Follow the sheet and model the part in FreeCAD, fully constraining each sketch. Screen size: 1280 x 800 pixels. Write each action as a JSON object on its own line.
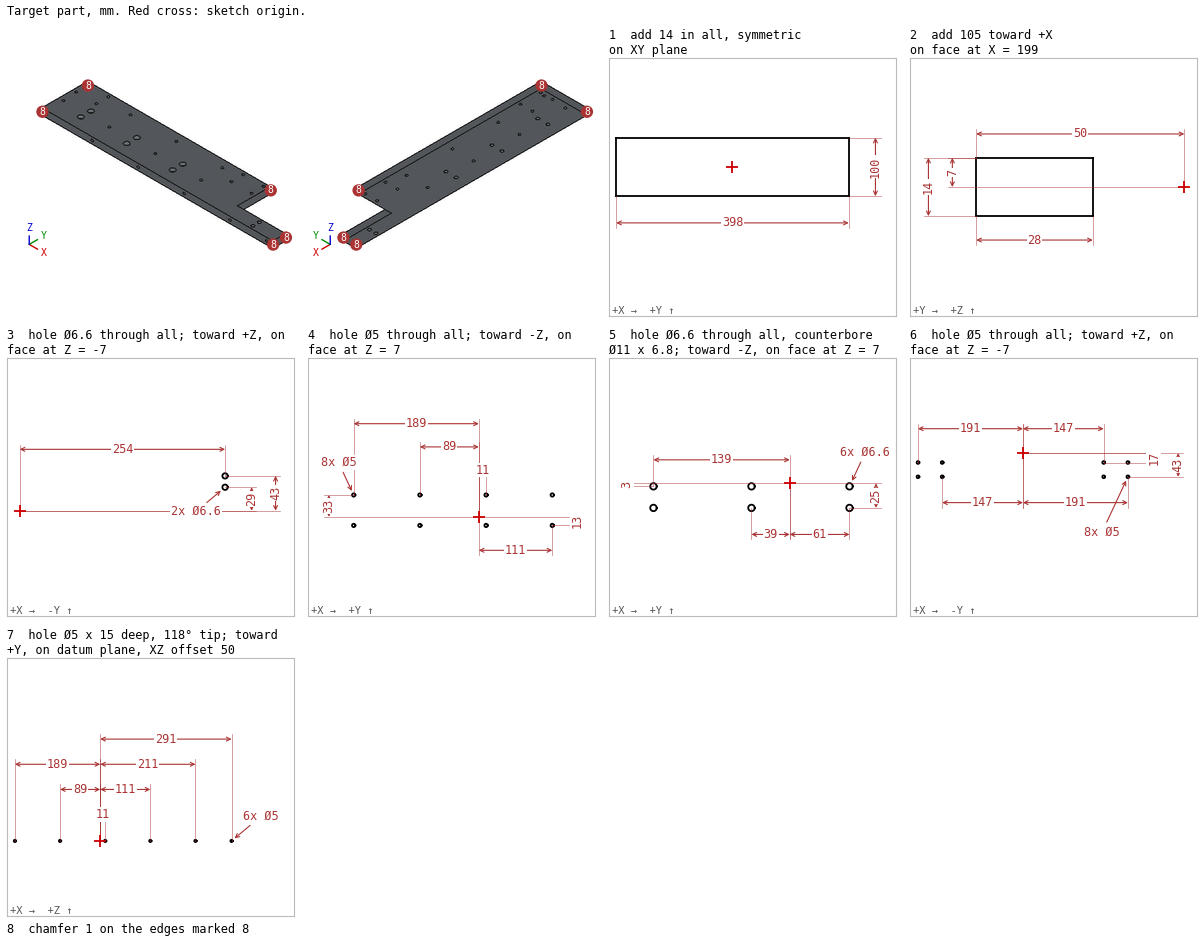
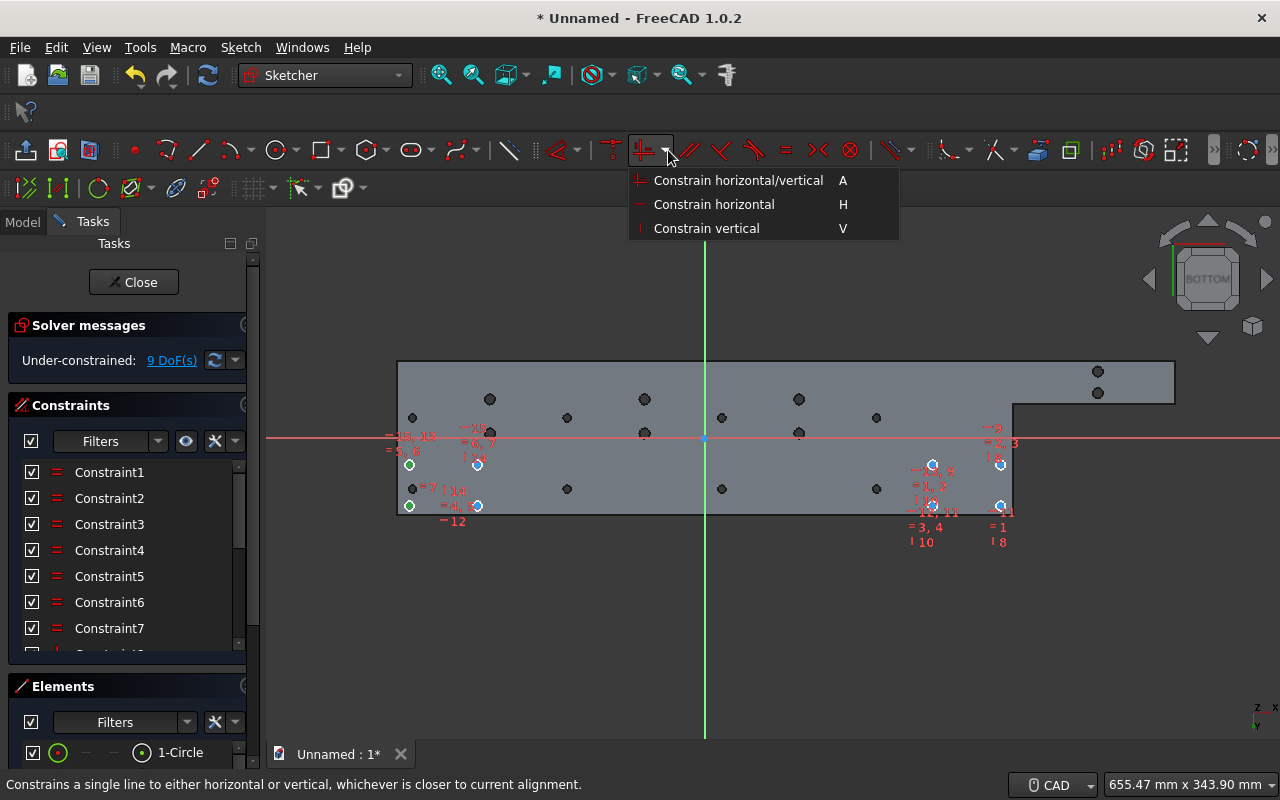
{"action": "left_click", "coordinate": [764, 228]}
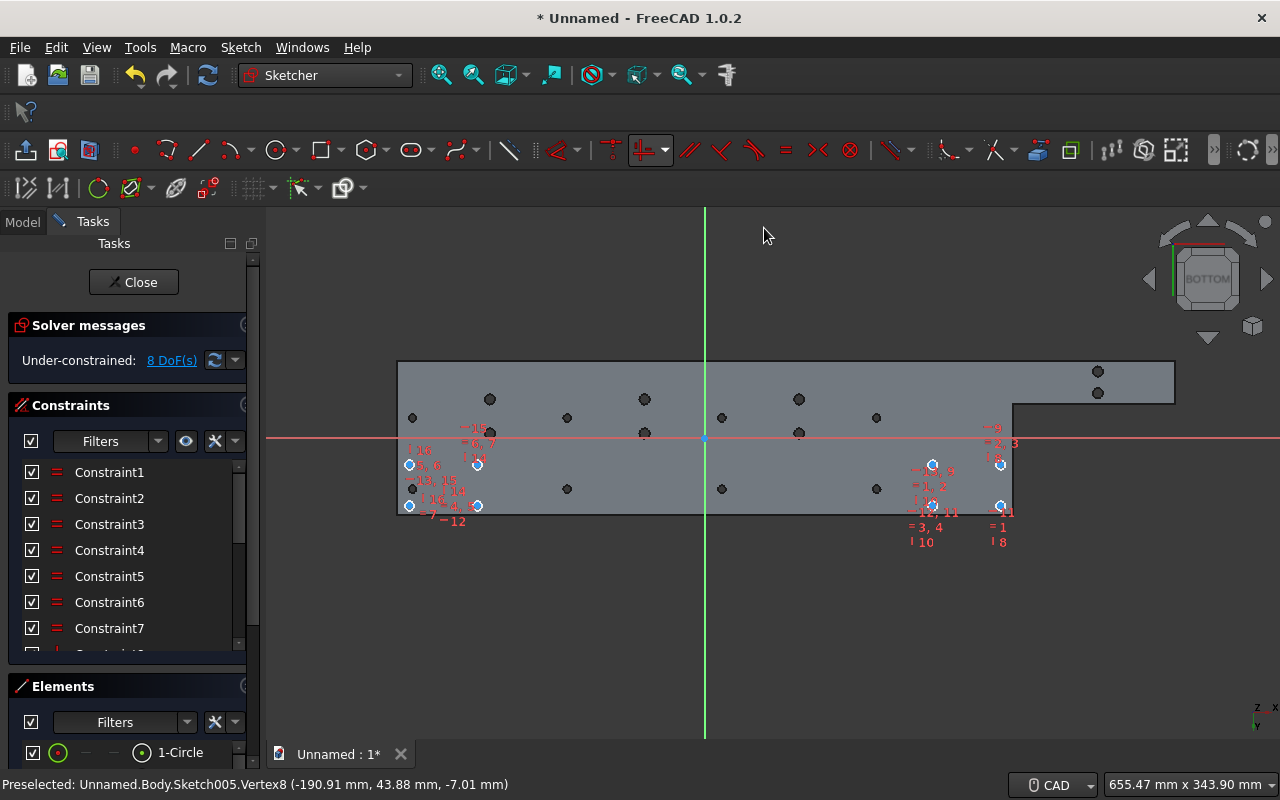
{"action": "left_click", "coordinate": [478, 506]}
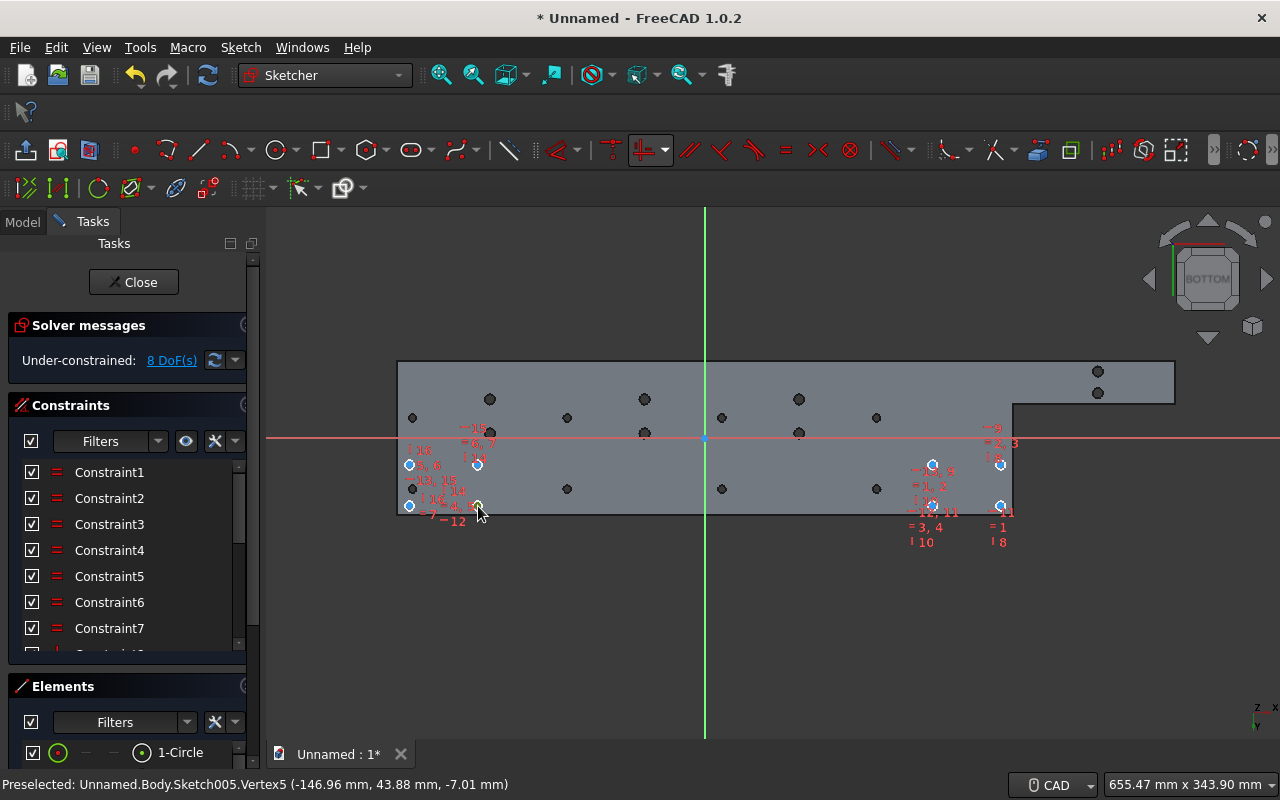
{"action": "left_click", "coordinate": [410, 506]}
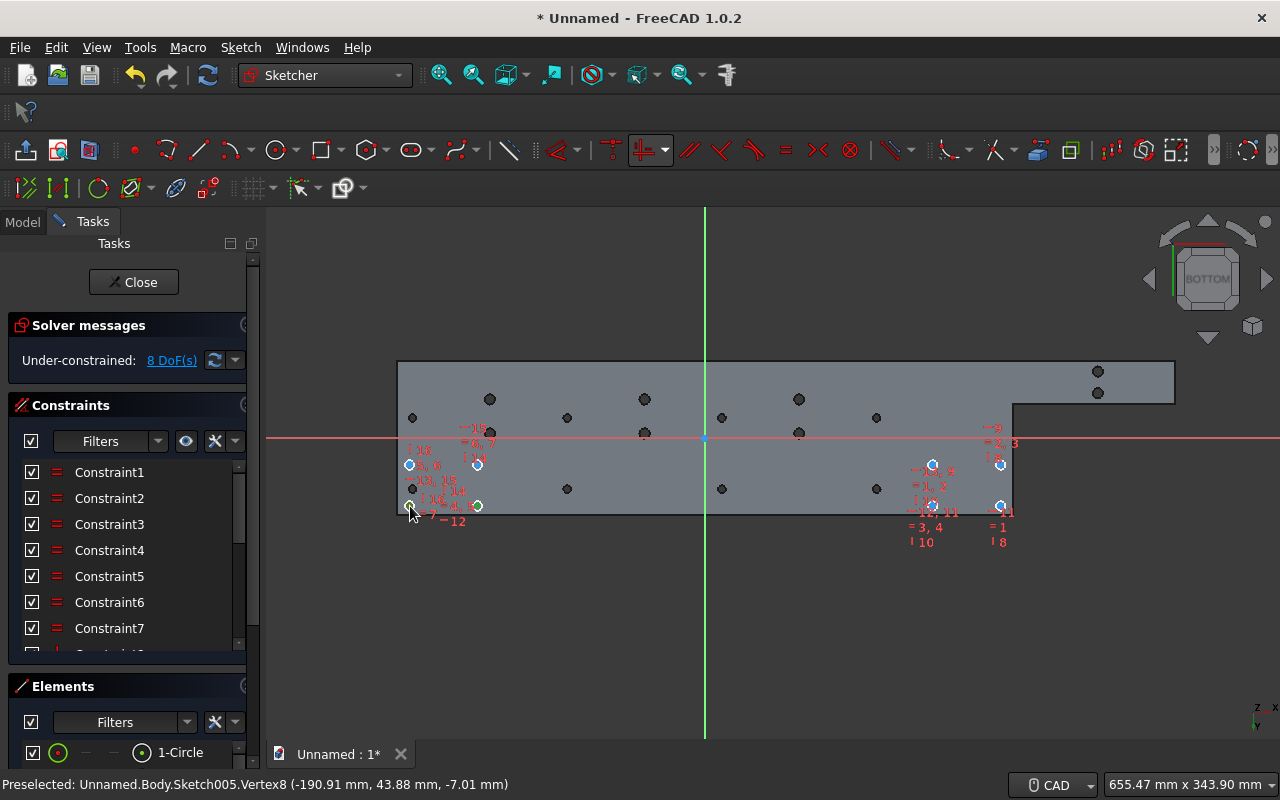
{"action": "key", "text": "h"}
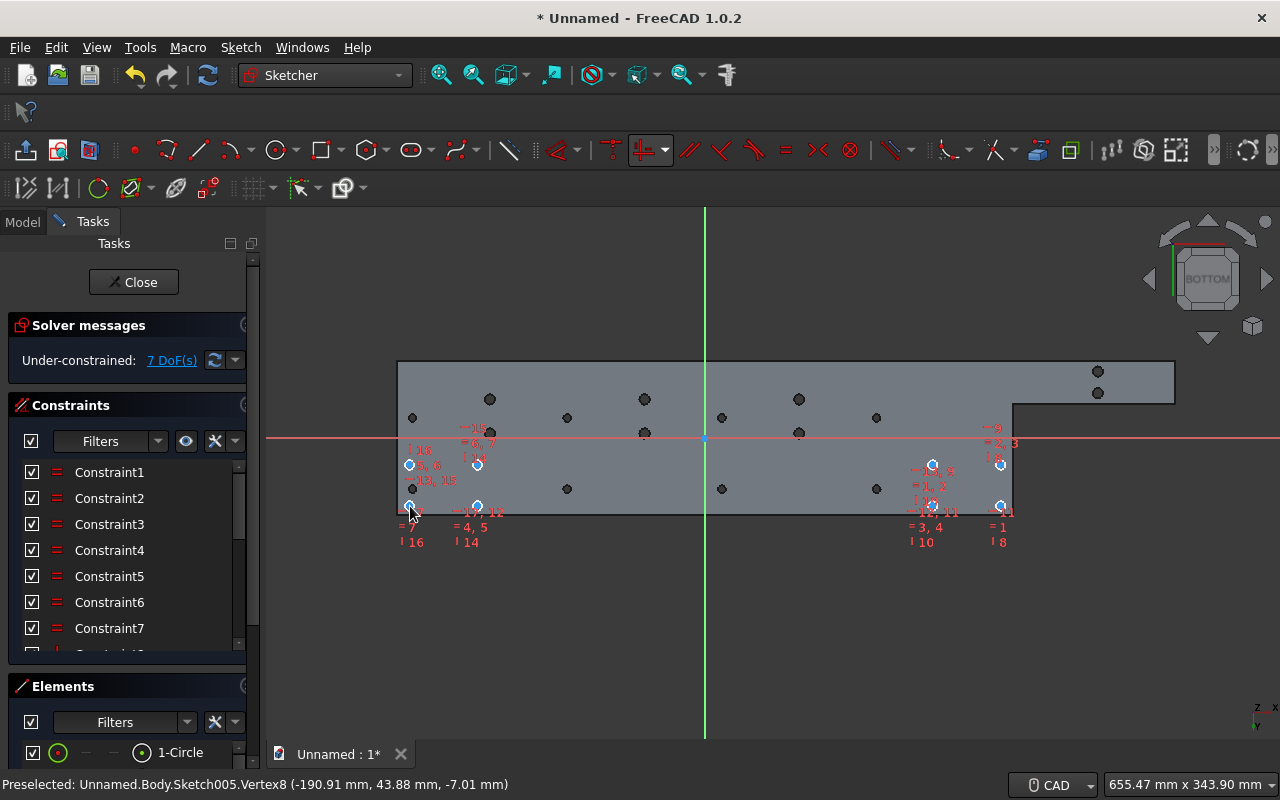
{"action": "key", "text": "d"}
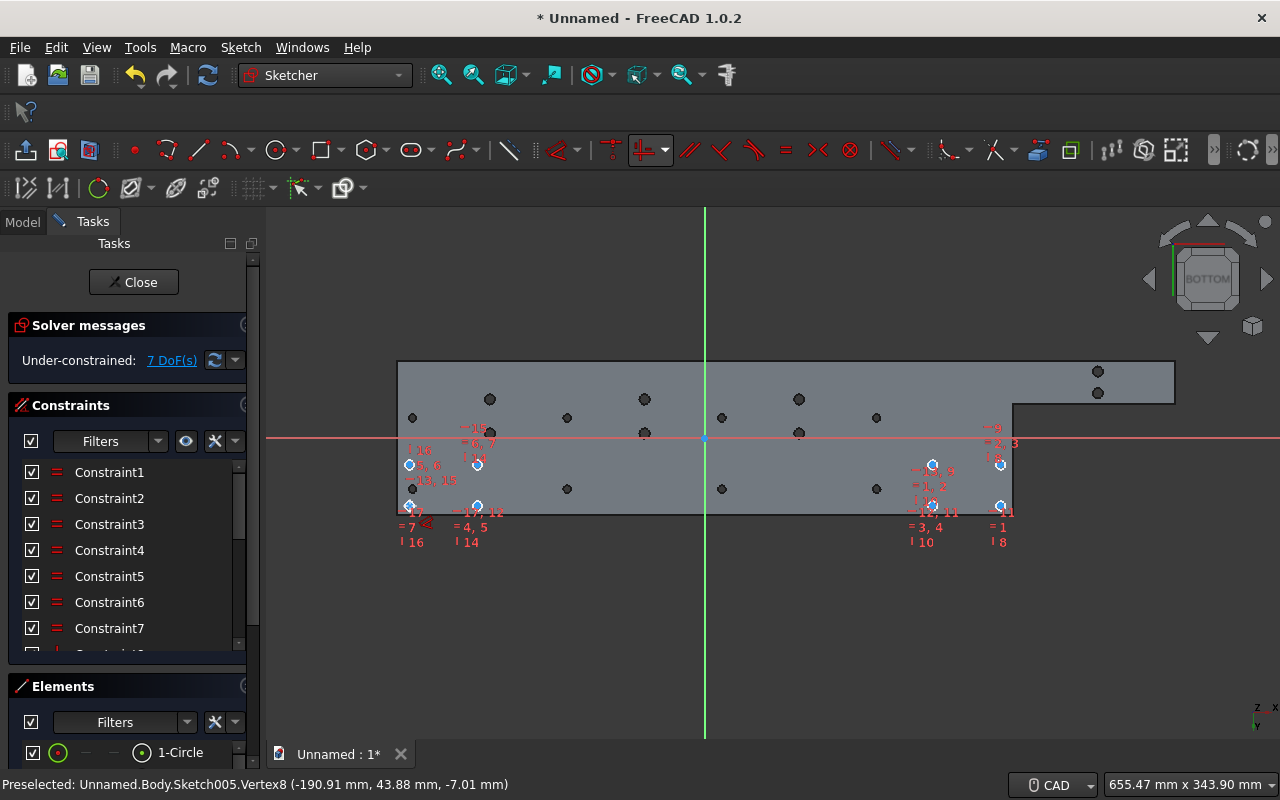
{"action": "scroll", "coordinate": [1004, 503], "scroll_direction": "up", "scroll_amount": 9}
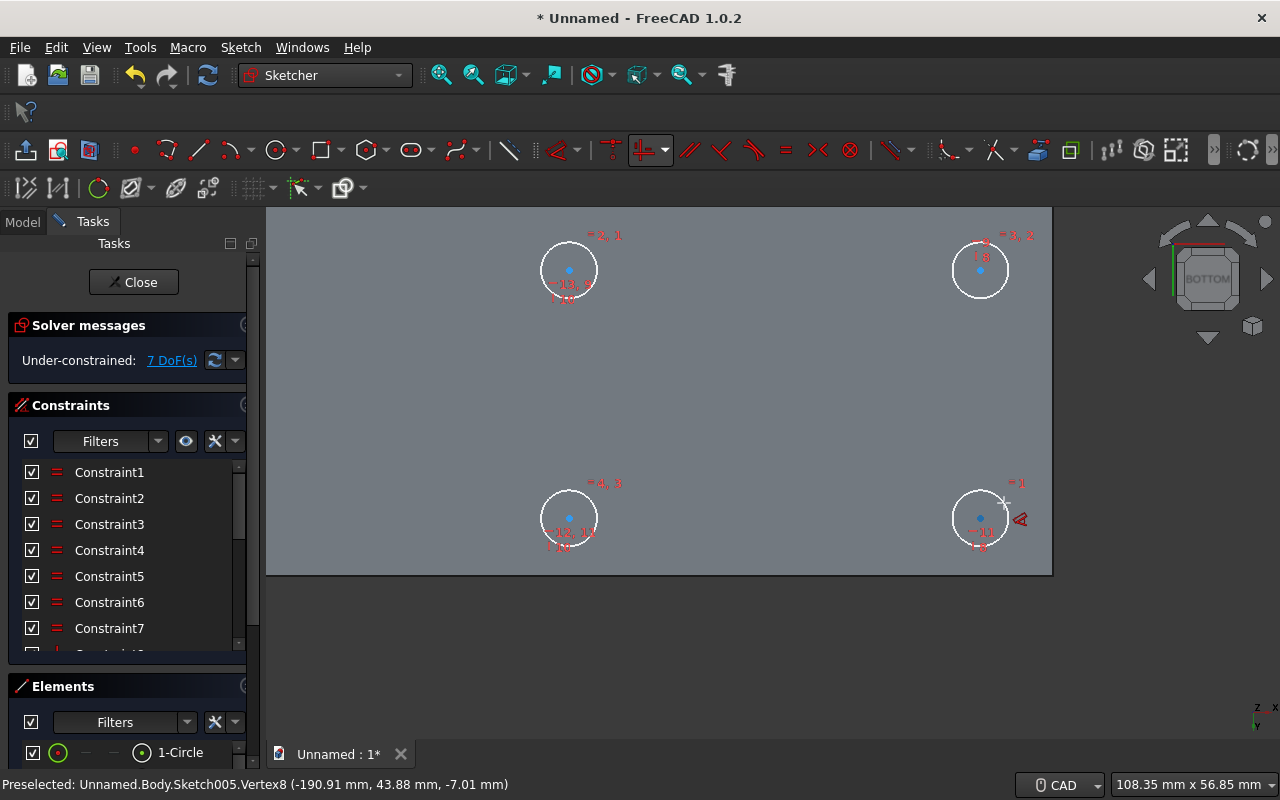
{"action": "left_click", "coordinate": [1000, 499]}
{"action": "left_click", "coordinate": [1023, 476]}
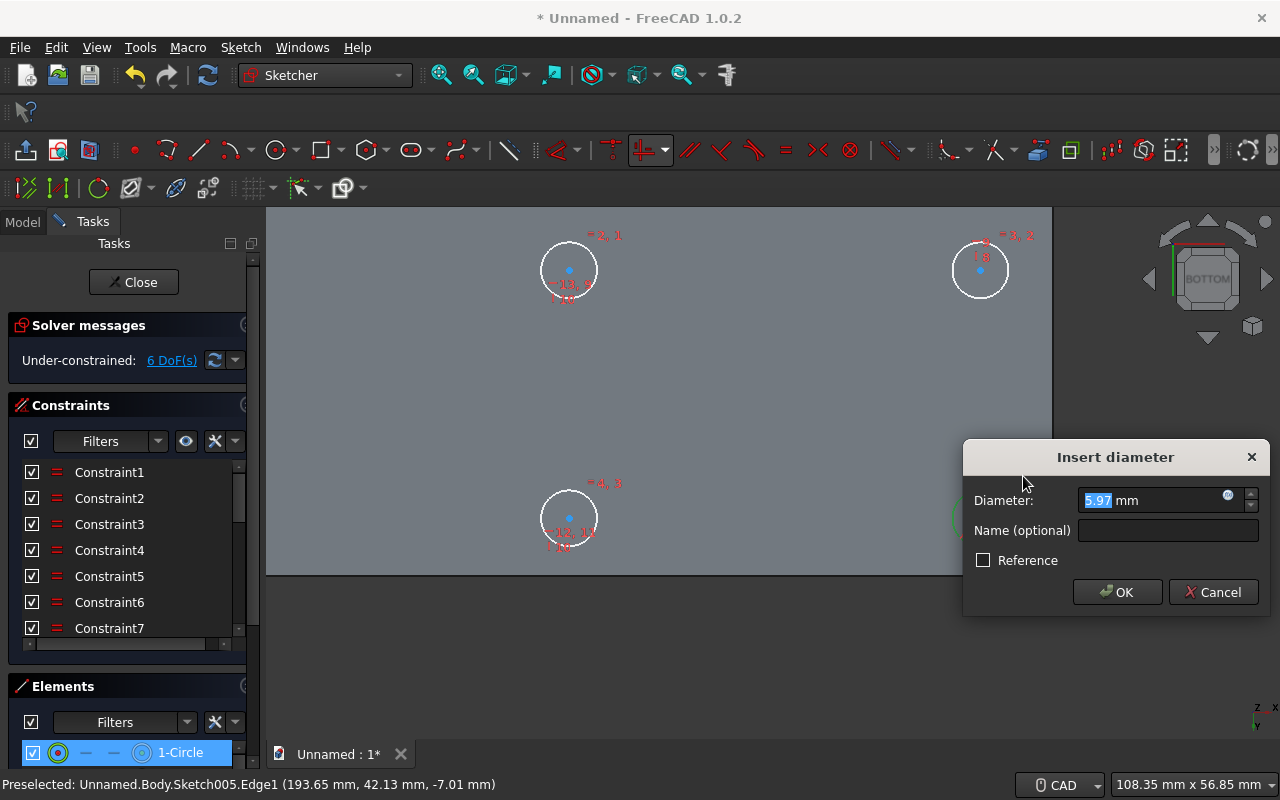
{"action": "type", "text": "5"}
{"action": "key", "text": "Return"}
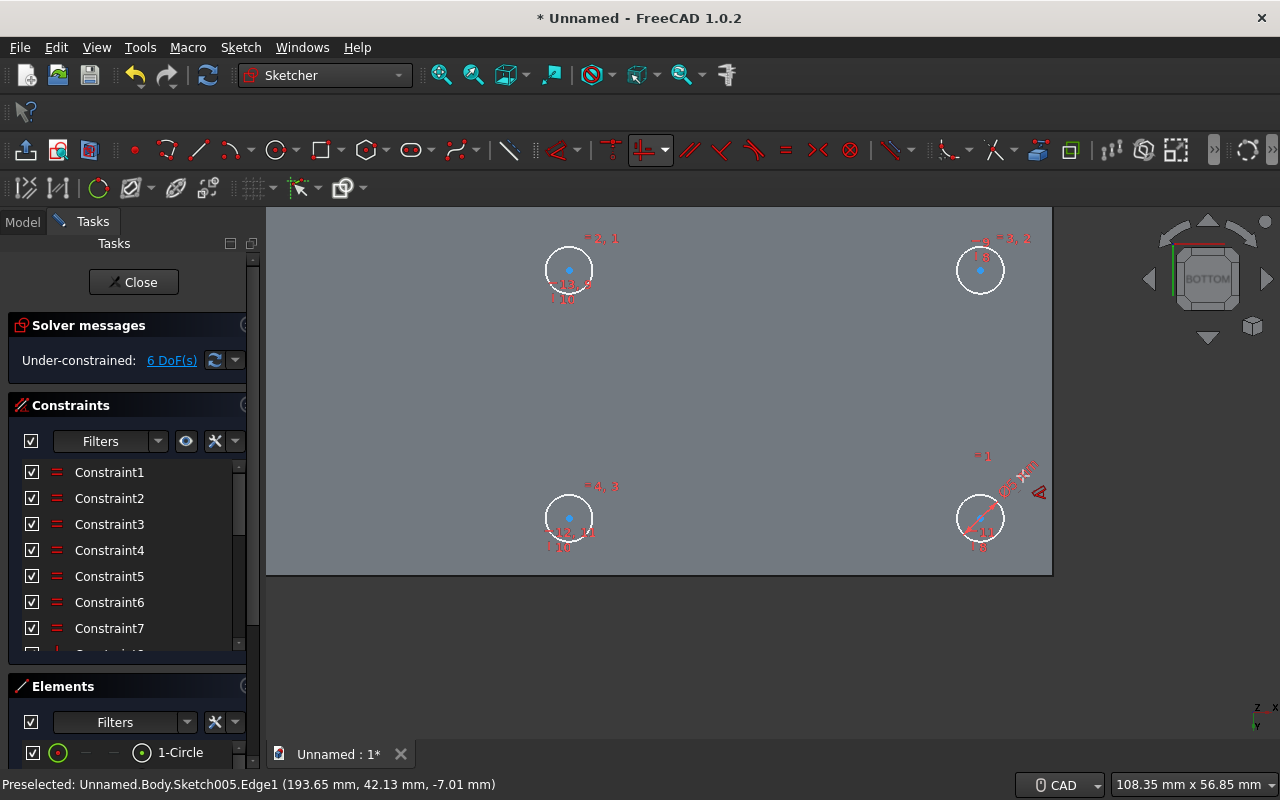
{"action": "scroll", "coordinate": [1004, 503], "scroll_direction": "down", "scroll_amount": 9}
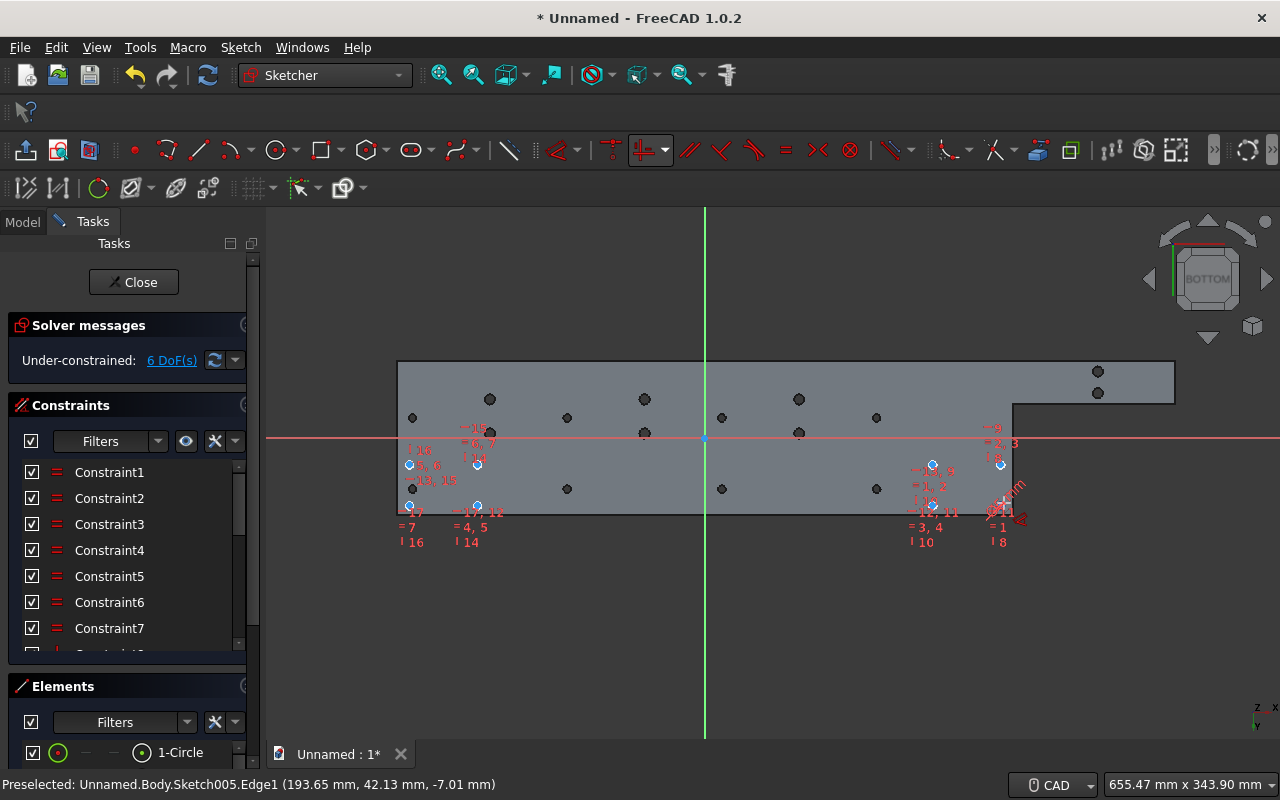
{"action": "left_click", "coordinate": [1001, 506]}
{"action": "left_click", "coordinate": [1035, 472]}